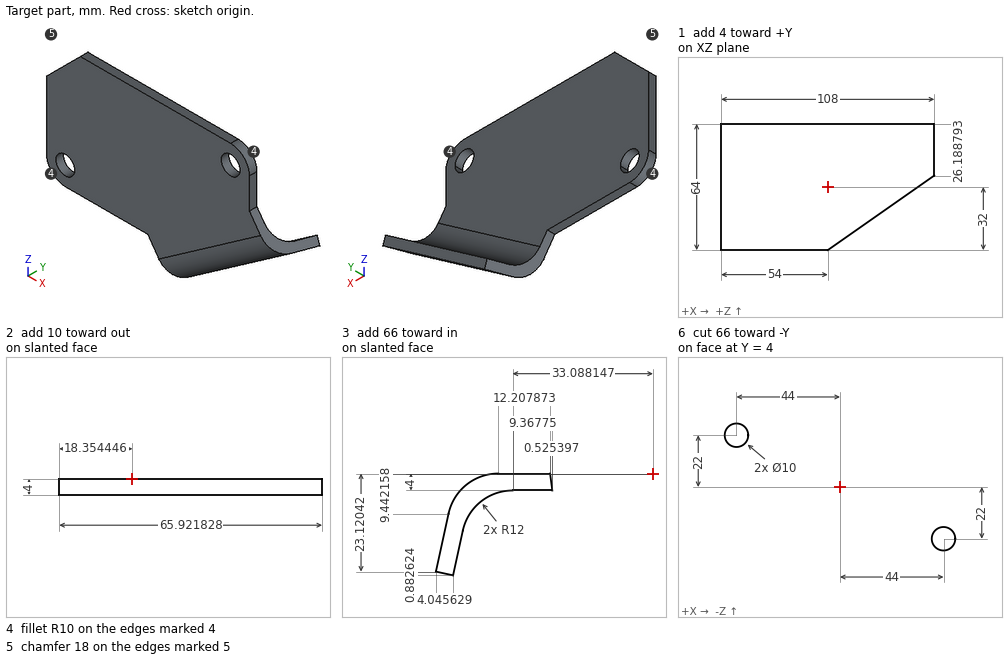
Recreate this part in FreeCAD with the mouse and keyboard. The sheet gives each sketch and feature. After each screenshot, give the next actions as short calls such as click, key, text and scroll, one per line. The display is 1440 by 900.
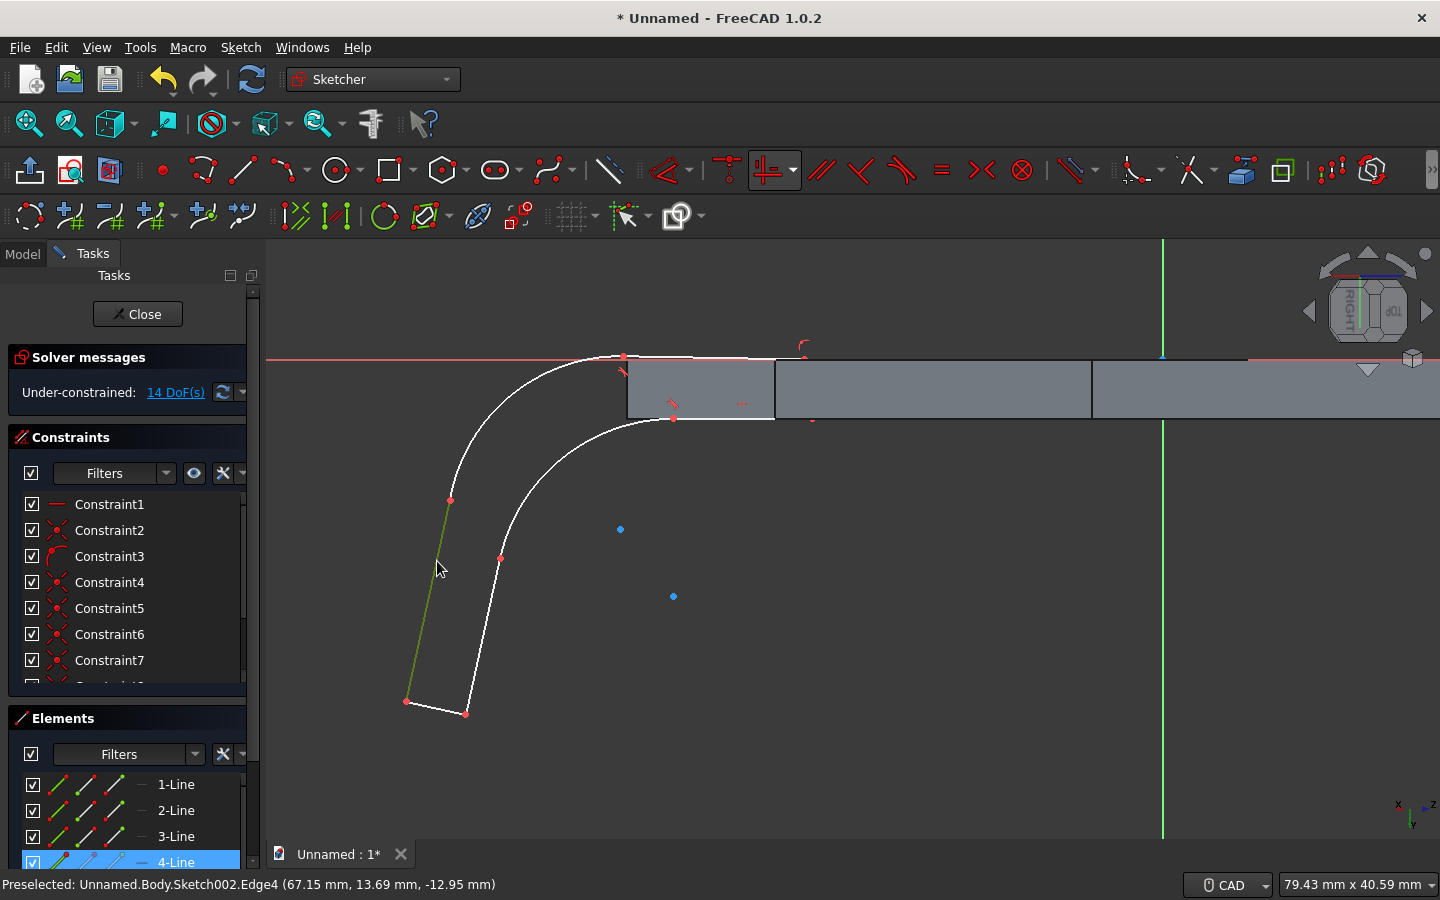
scroll(552, 370, up, 2)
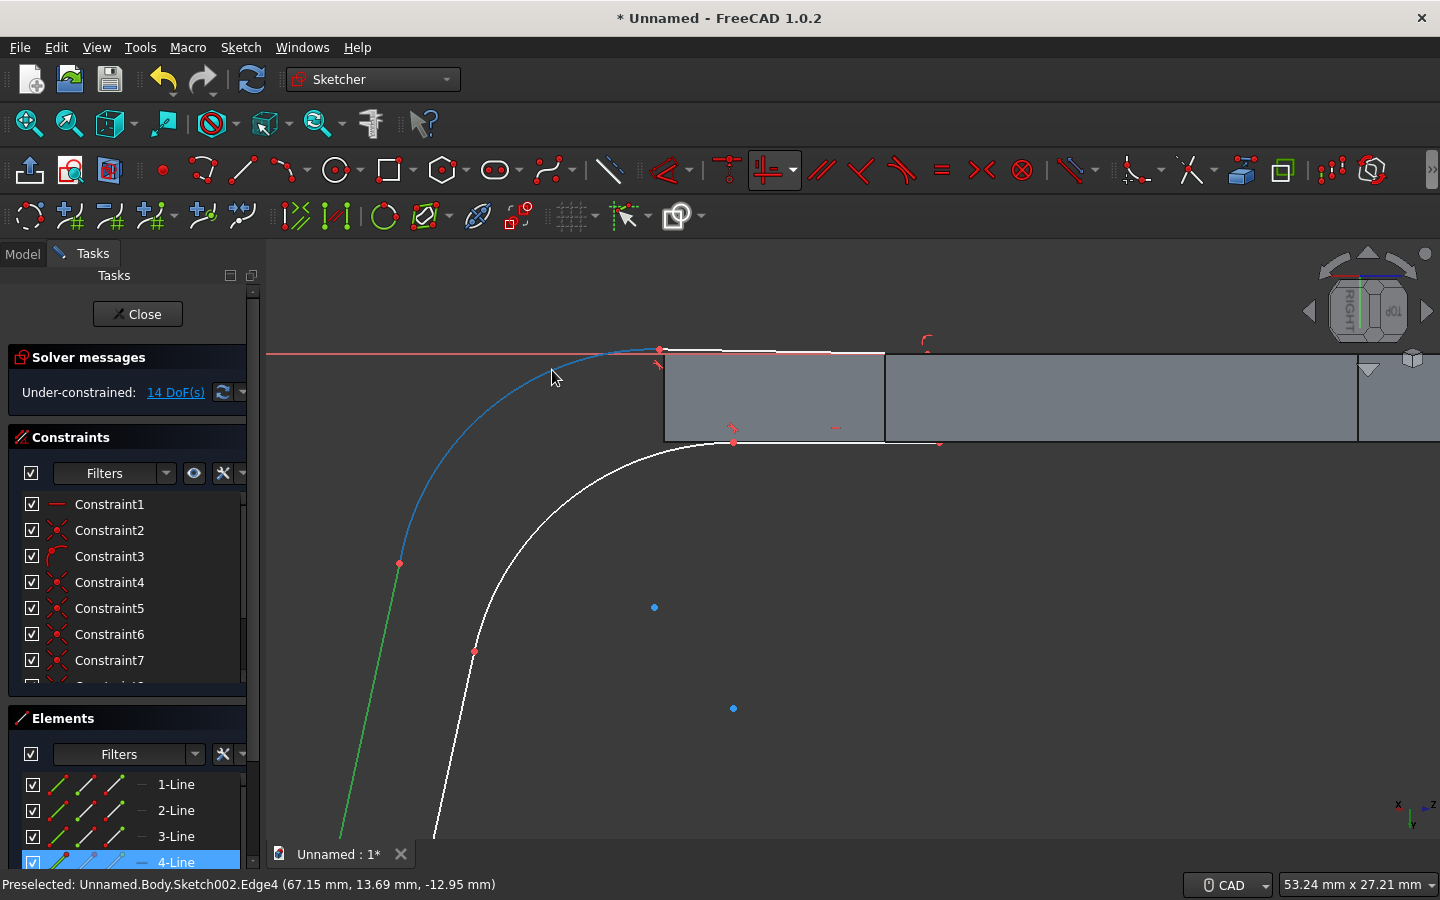
click(552, 370)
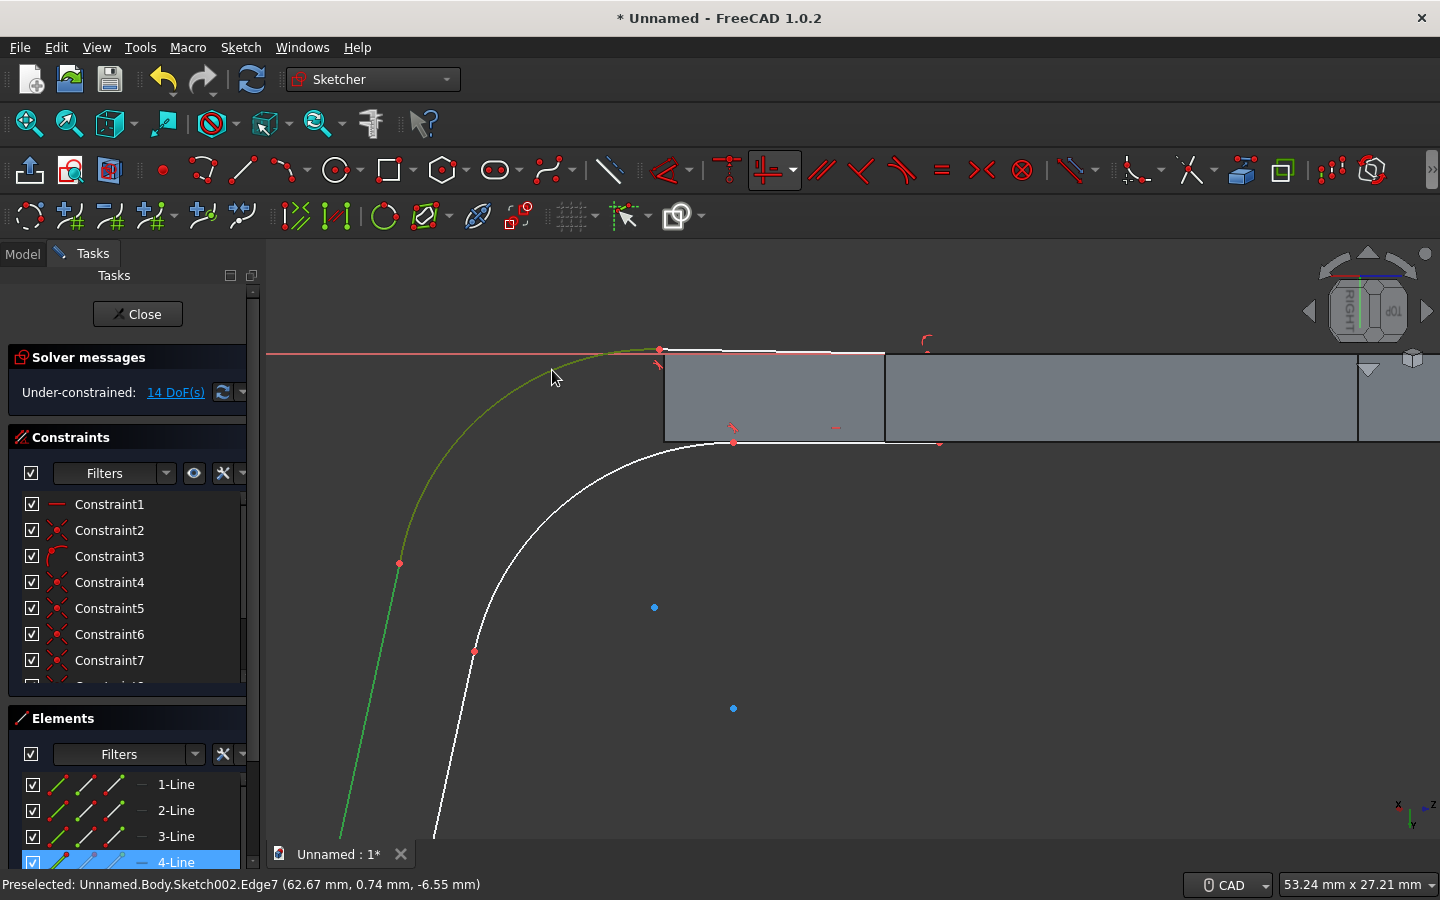
key(t)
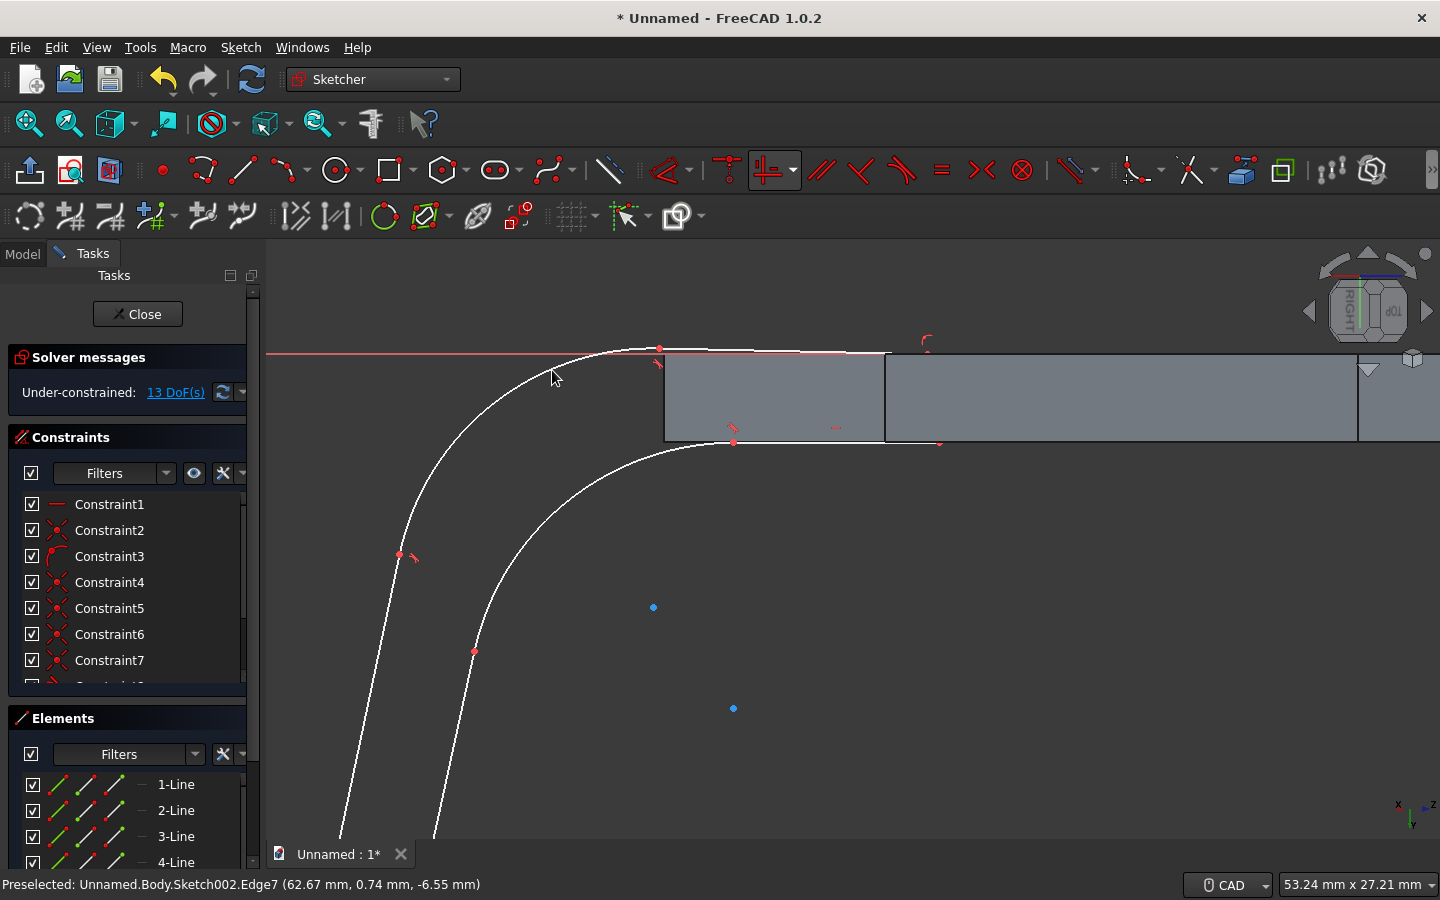
click(459, 722)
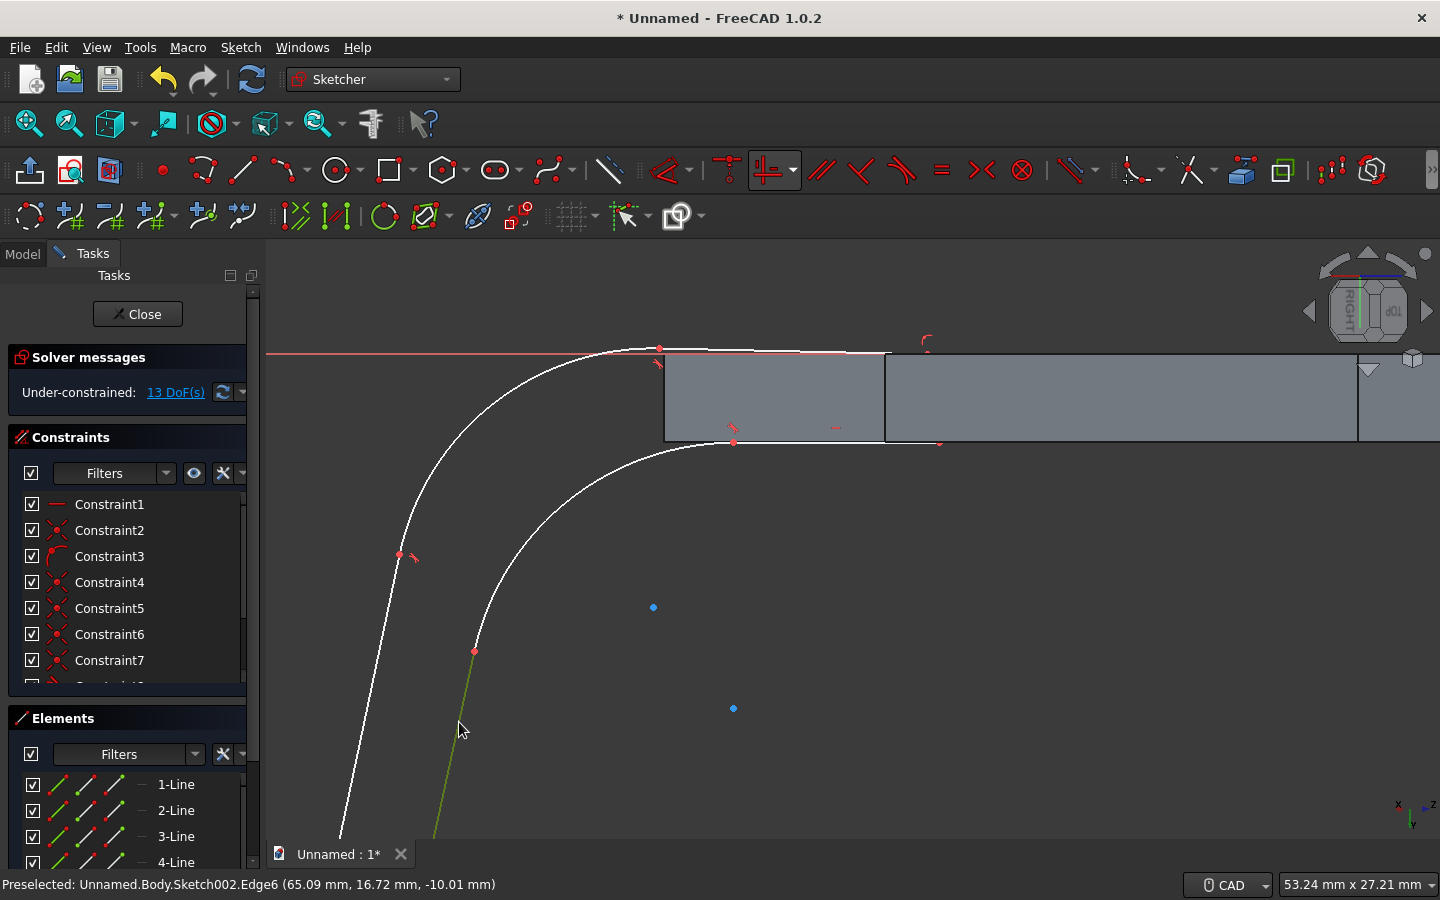
click(629, 464)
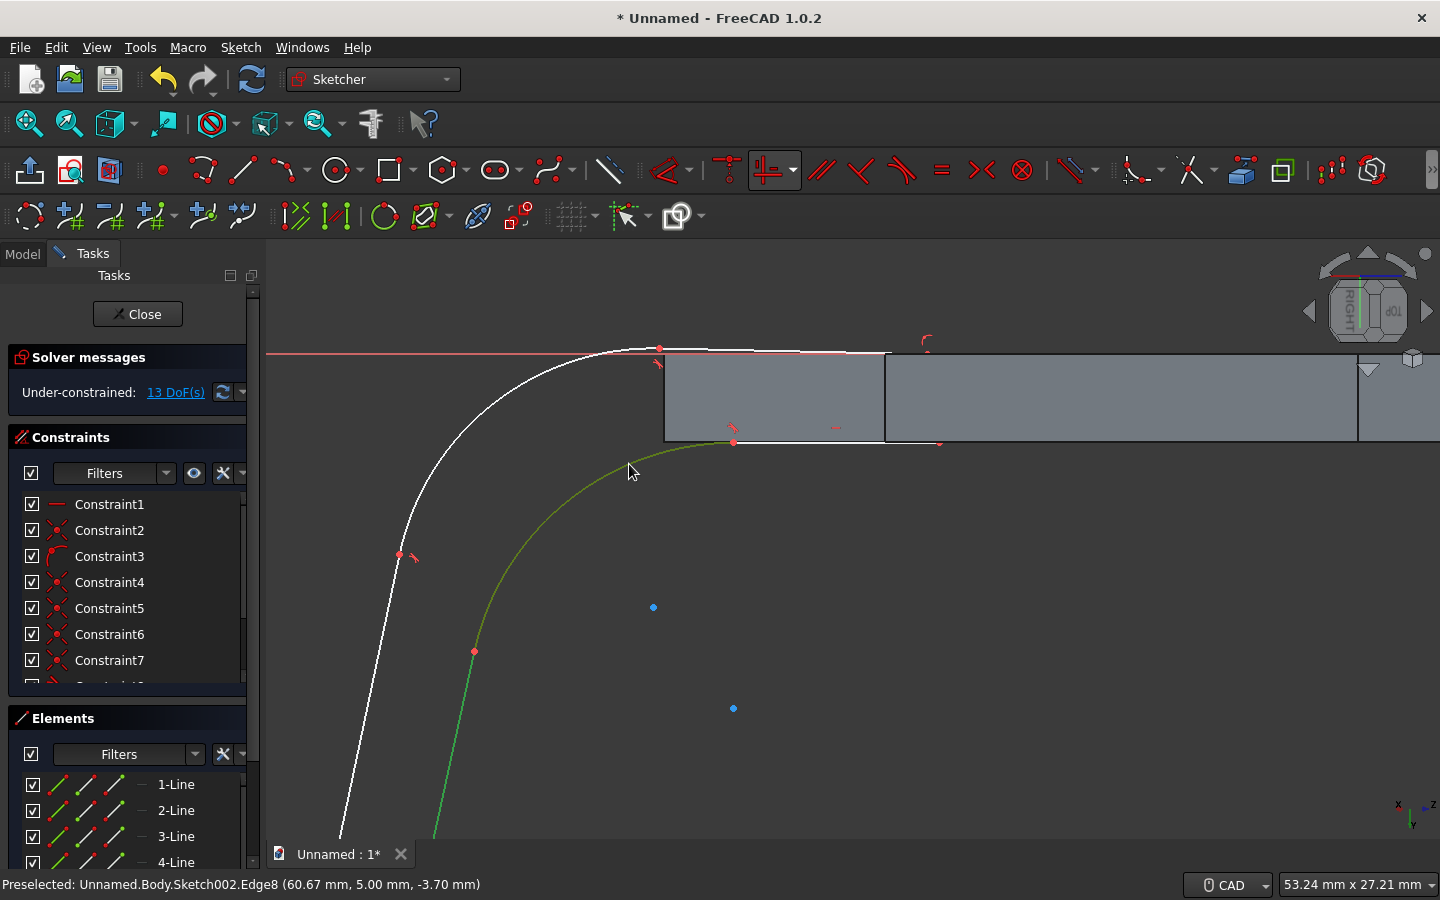
click(902, 170)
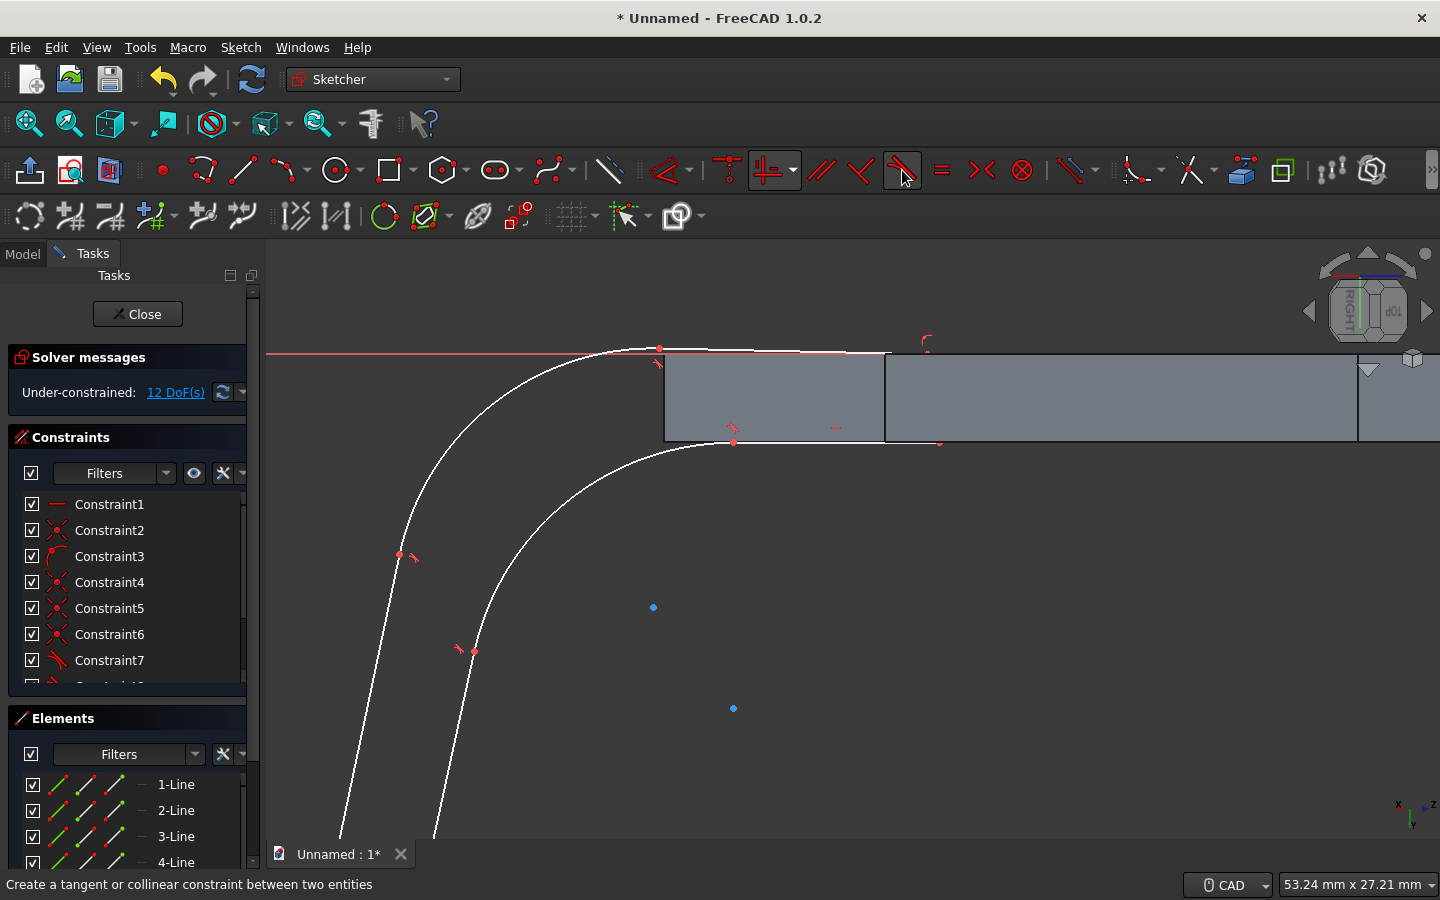
click(847, 353)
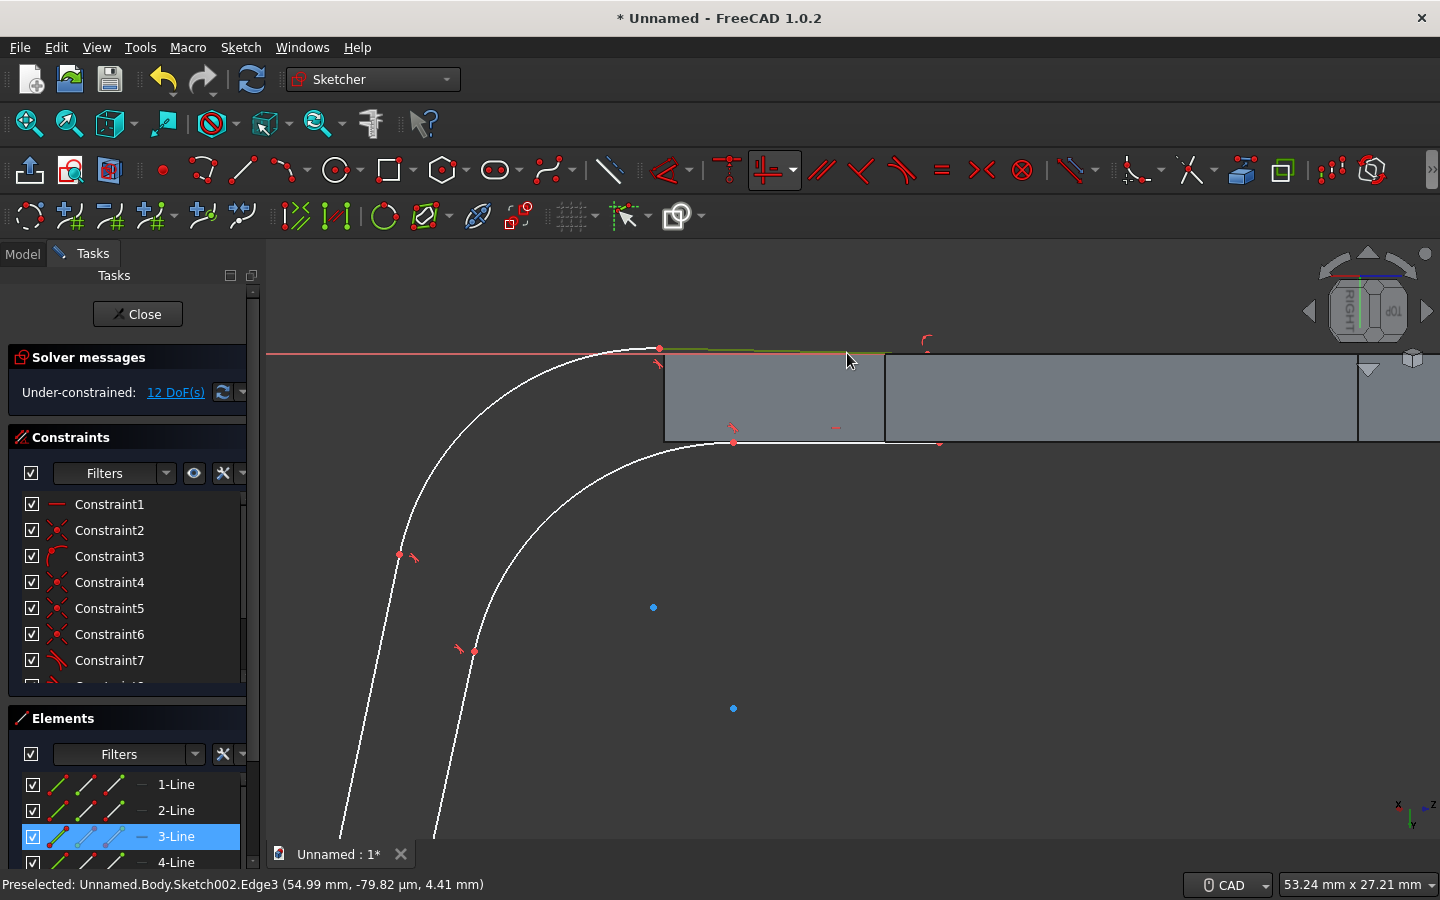
key(h)